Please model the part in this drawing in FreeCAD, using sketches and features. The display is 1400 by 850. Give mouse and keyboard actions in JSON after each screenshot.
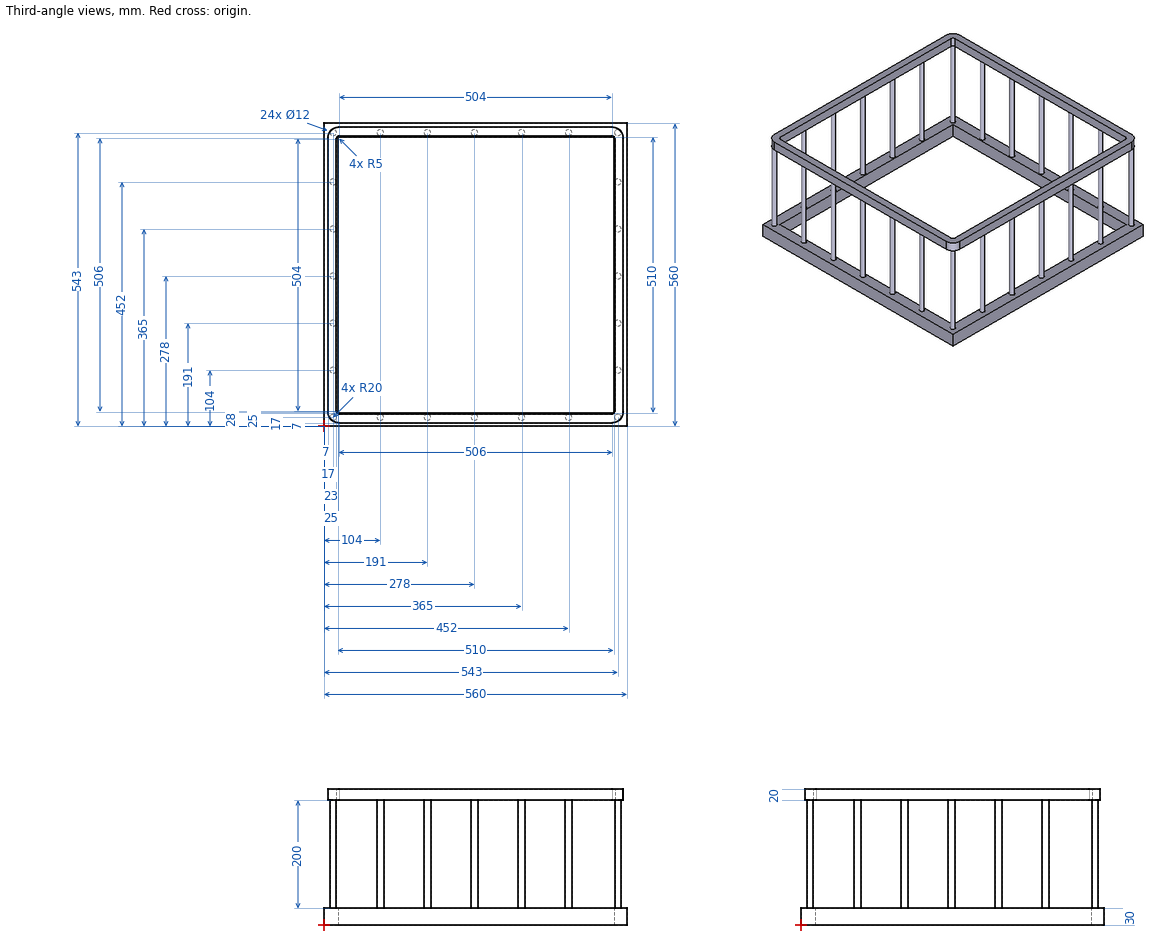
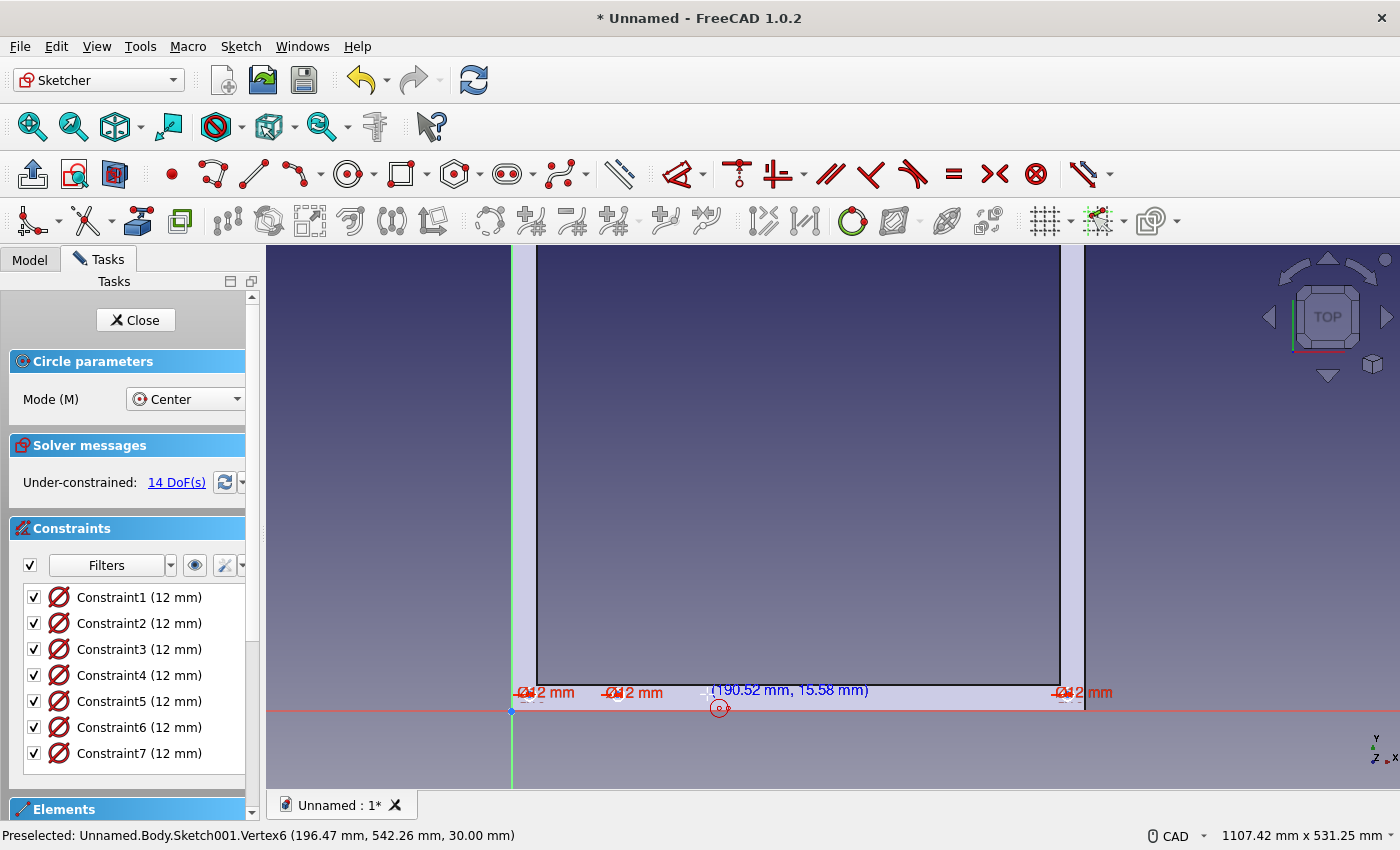
{"action": "left_click", "coordinate": [707, 694]}
{"action": "mouse_move", "coordinate": [712, 689]}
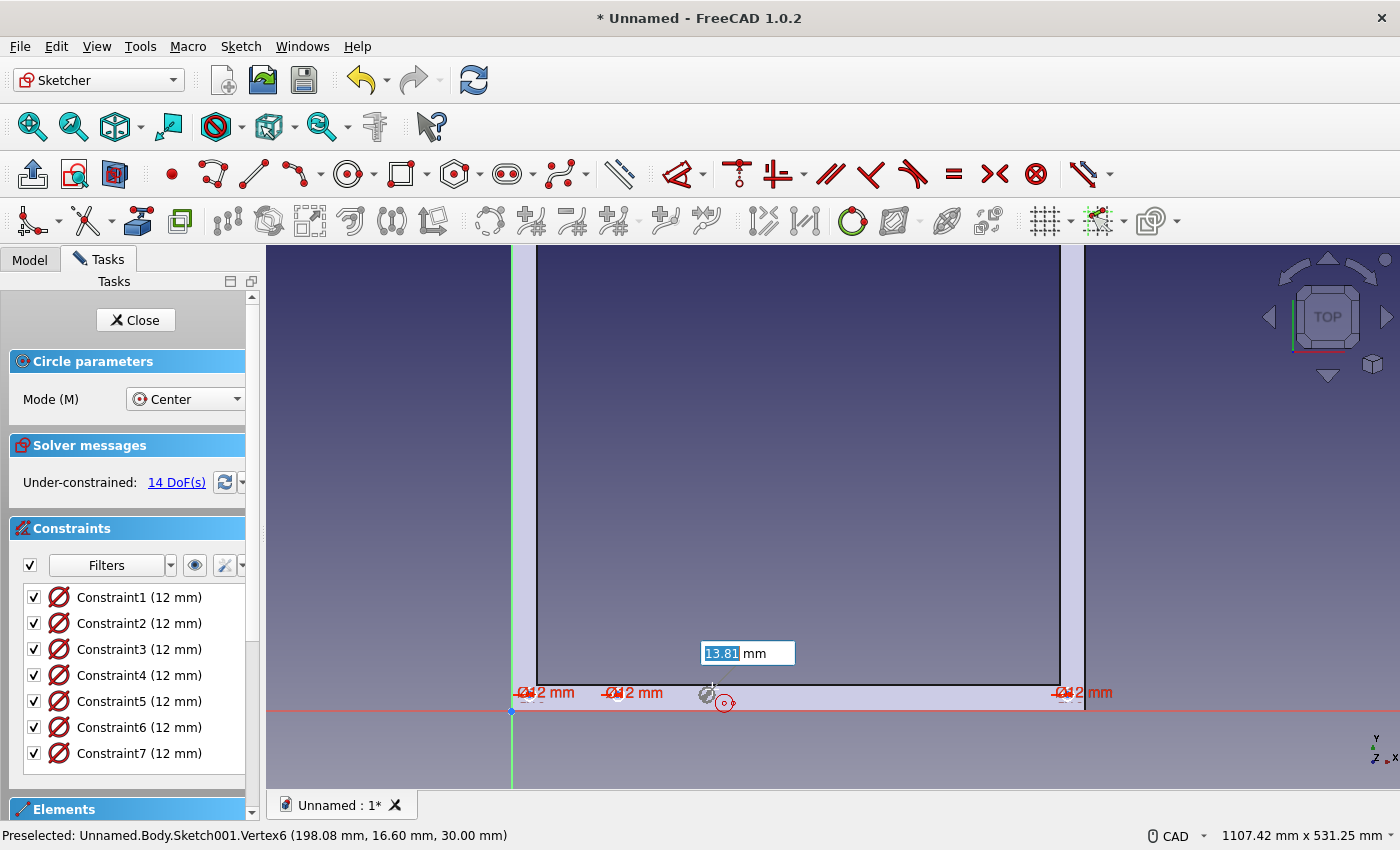
{"action": "type", "text": "12"}
{"action": "key", "text": "Return"}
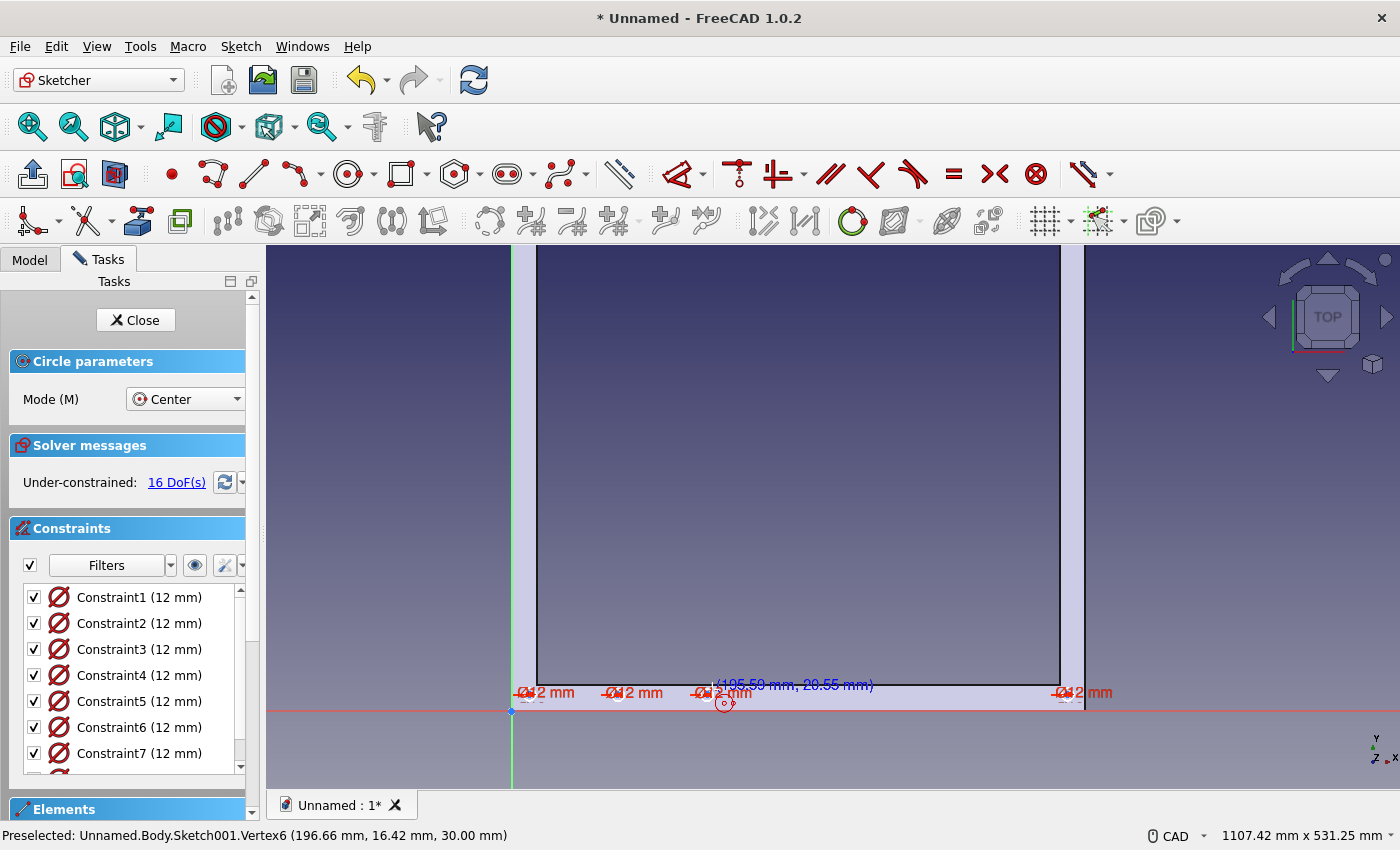
{"action": "scroll", "coordinate": [707, 694], "scroll_direction": "down", "scroll_amount": 2}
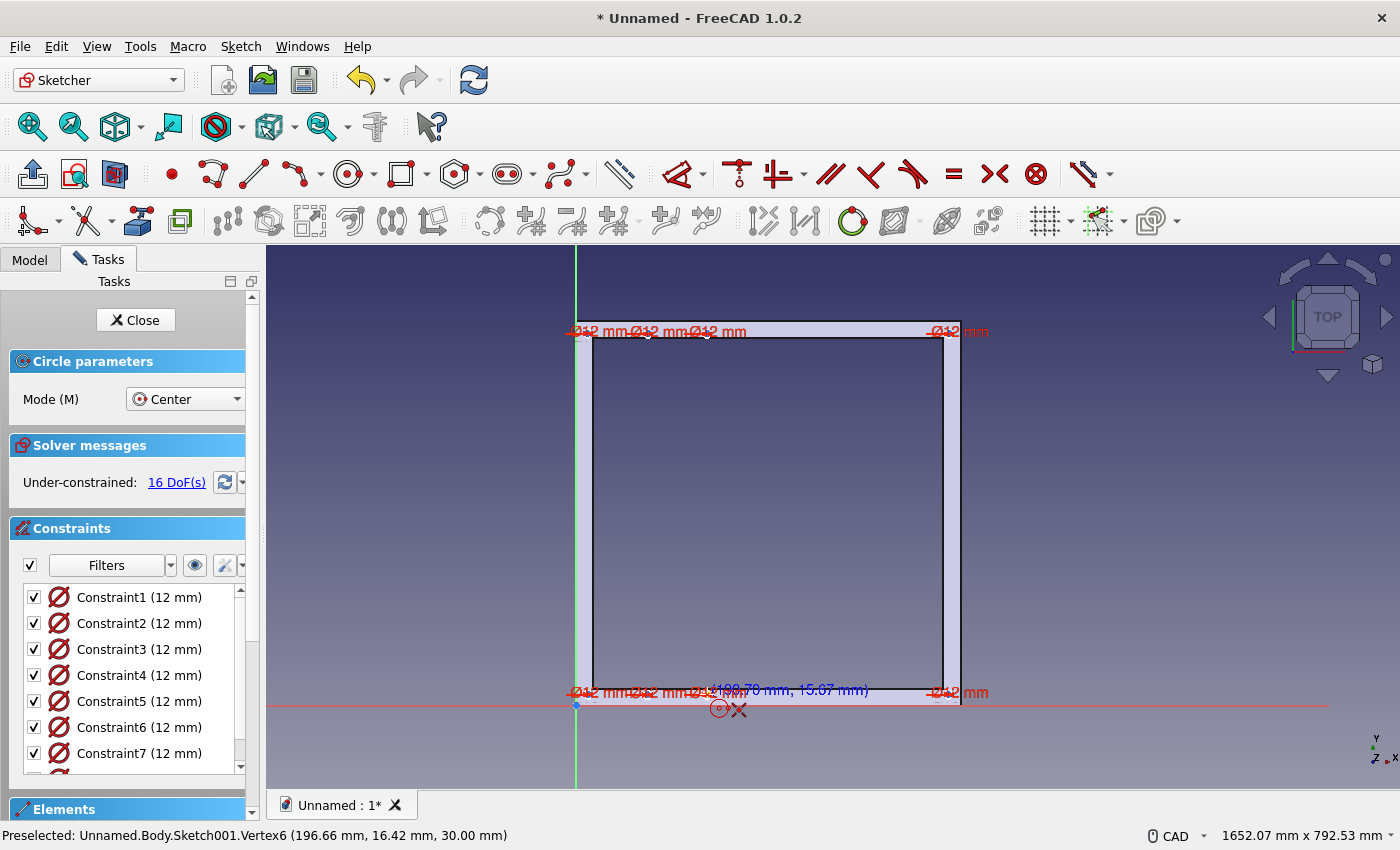
{"action": "scroll", "coordinate": [767, 333], "scroll_direction": "up", "scroll_amount": 9}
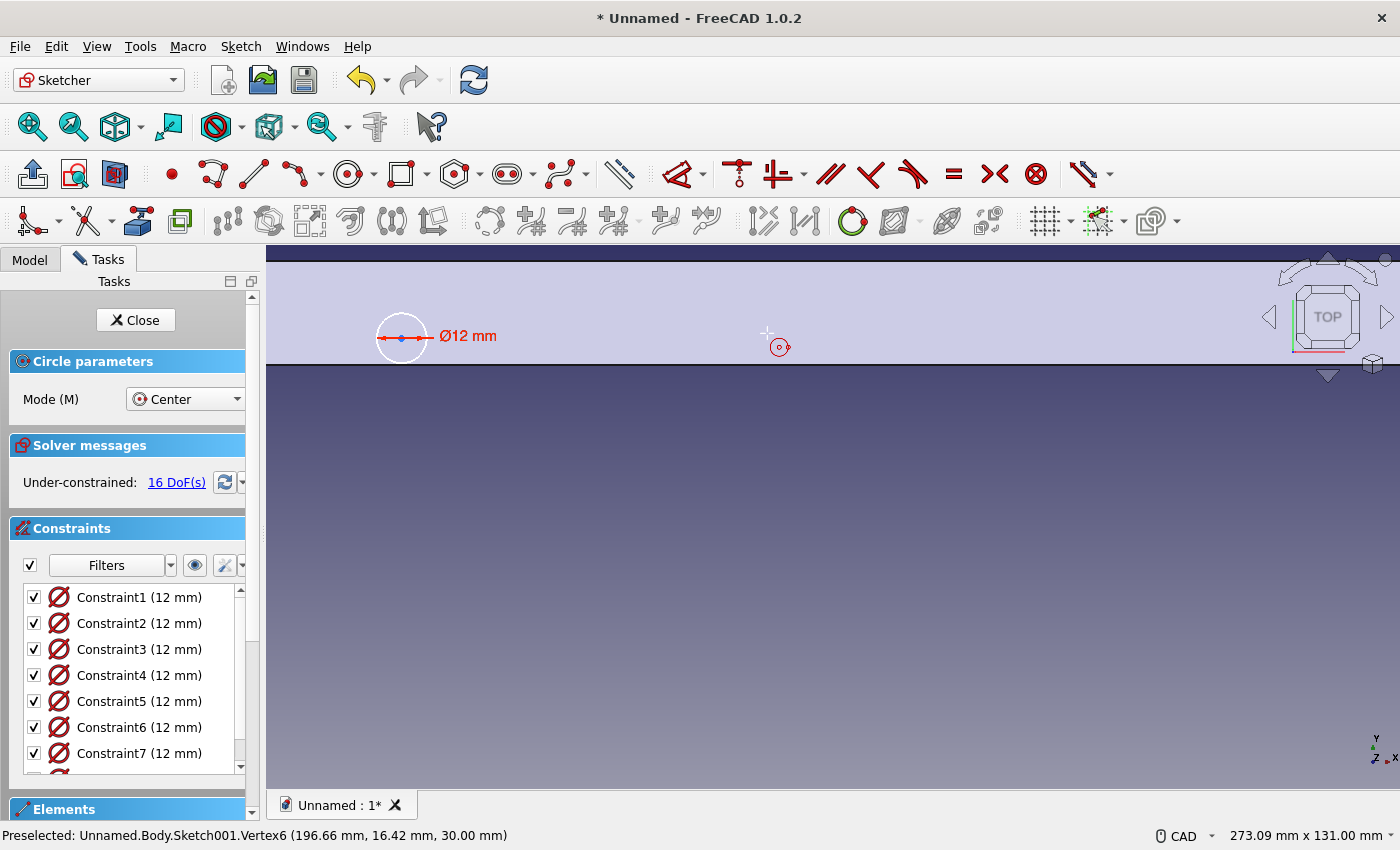
{"action": "scroll", "coordinate": [767, 333], "scroll_direction": "down", "scroll_amount": 9}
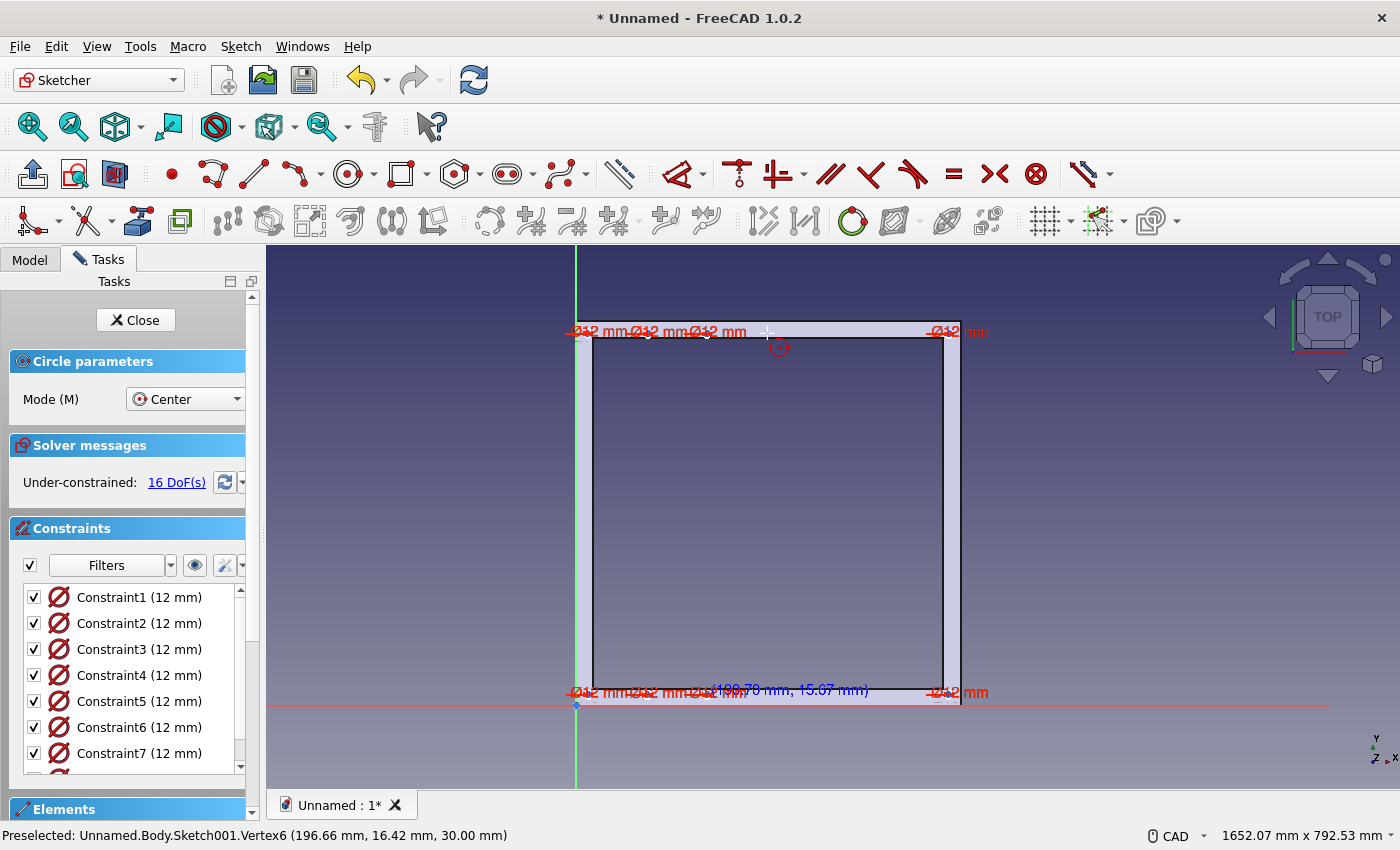
{"action": "left_click", "coordinate": [767, 333]}
{"action": "mouse_move", "coordinate": [770, 330]}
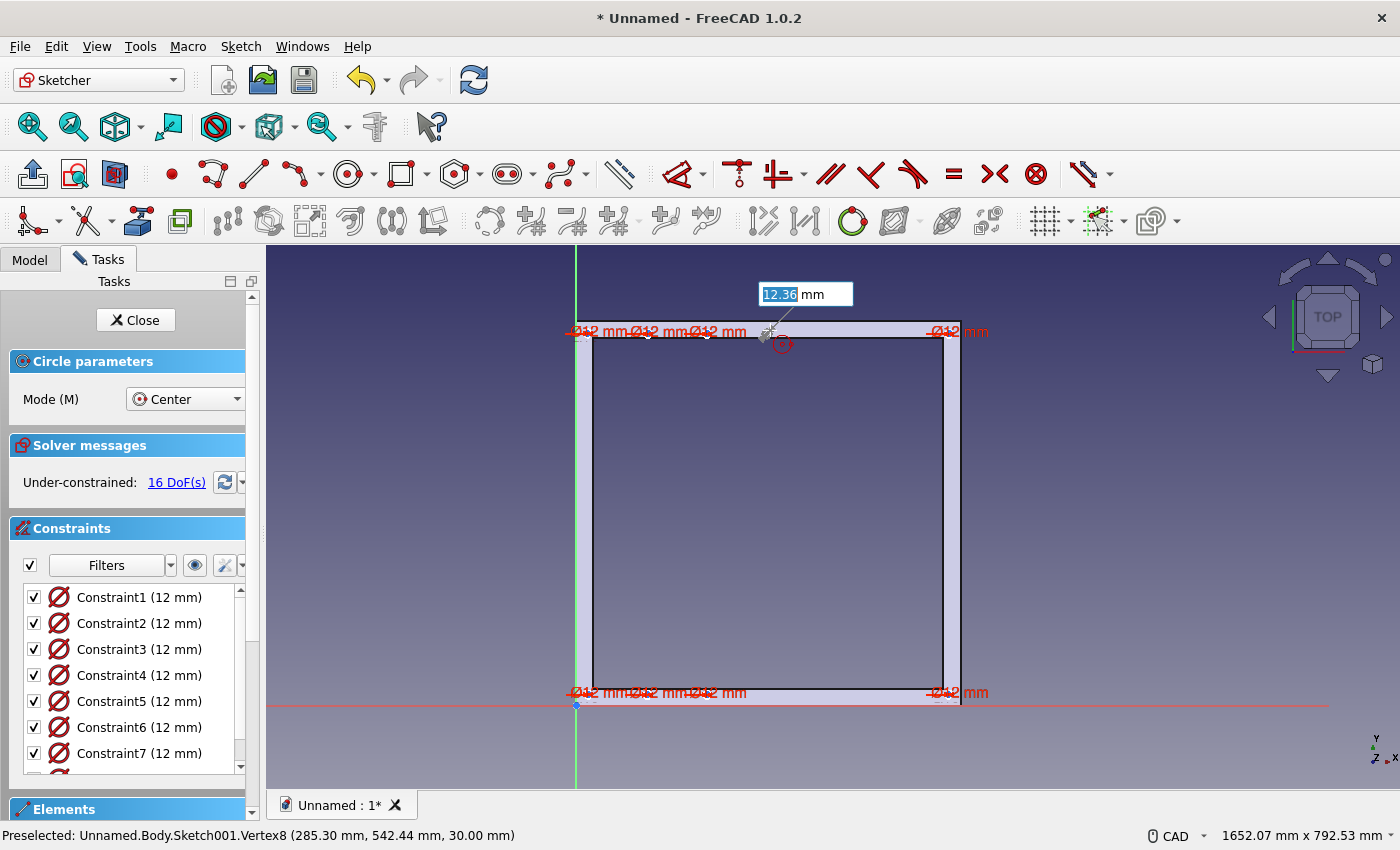
{"action": "type", "text": "12"}
{"action": "key", "text": "Return"}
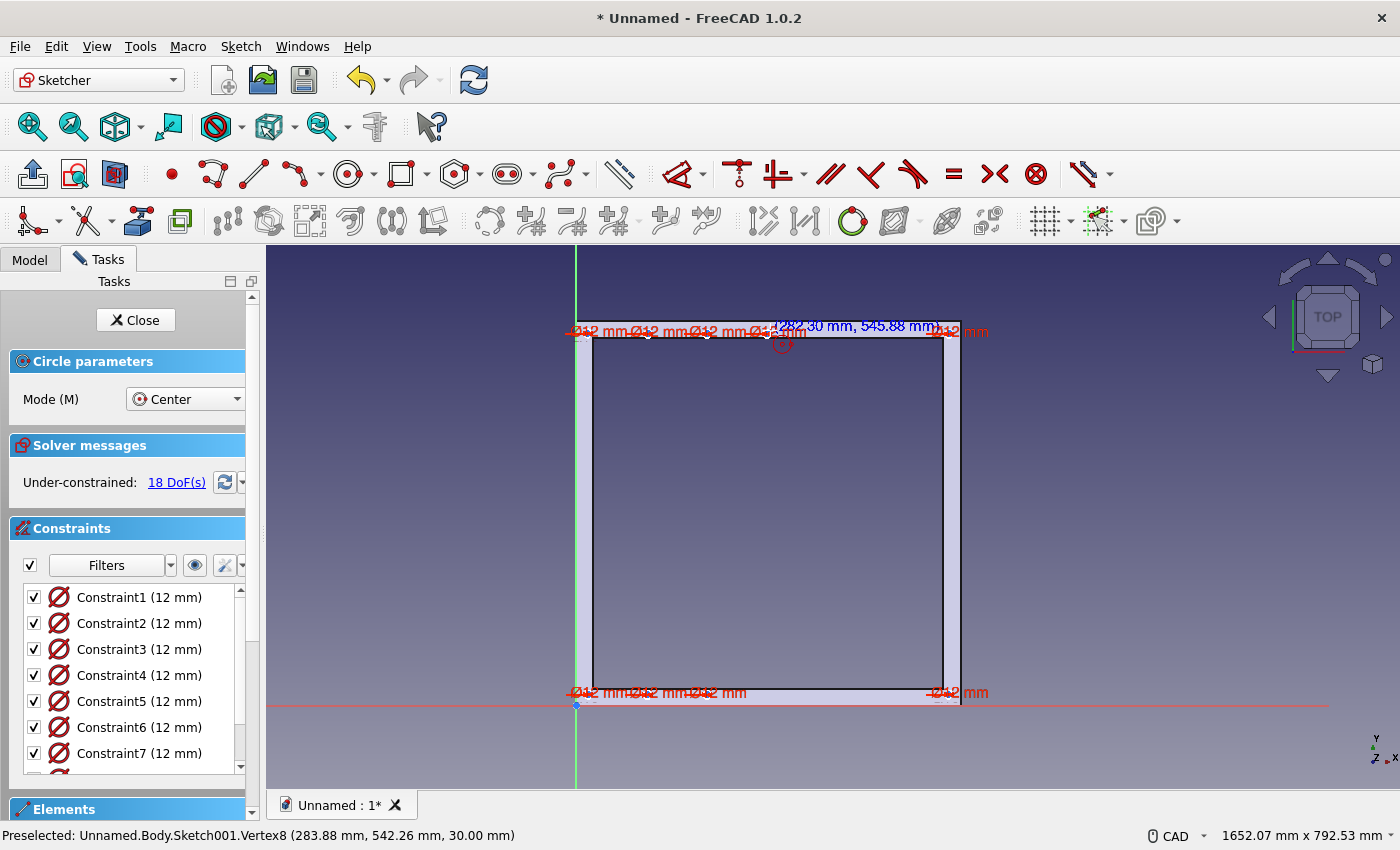
{"action": "scroll", "coordinate": [767, 694], "scroll_direction": "up", "scroll_amount": 9}